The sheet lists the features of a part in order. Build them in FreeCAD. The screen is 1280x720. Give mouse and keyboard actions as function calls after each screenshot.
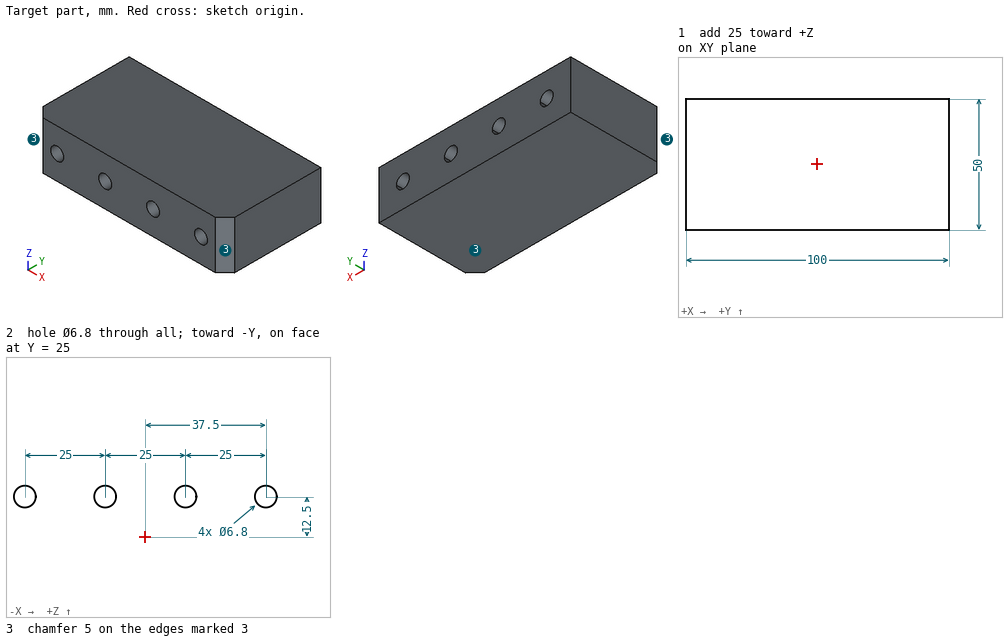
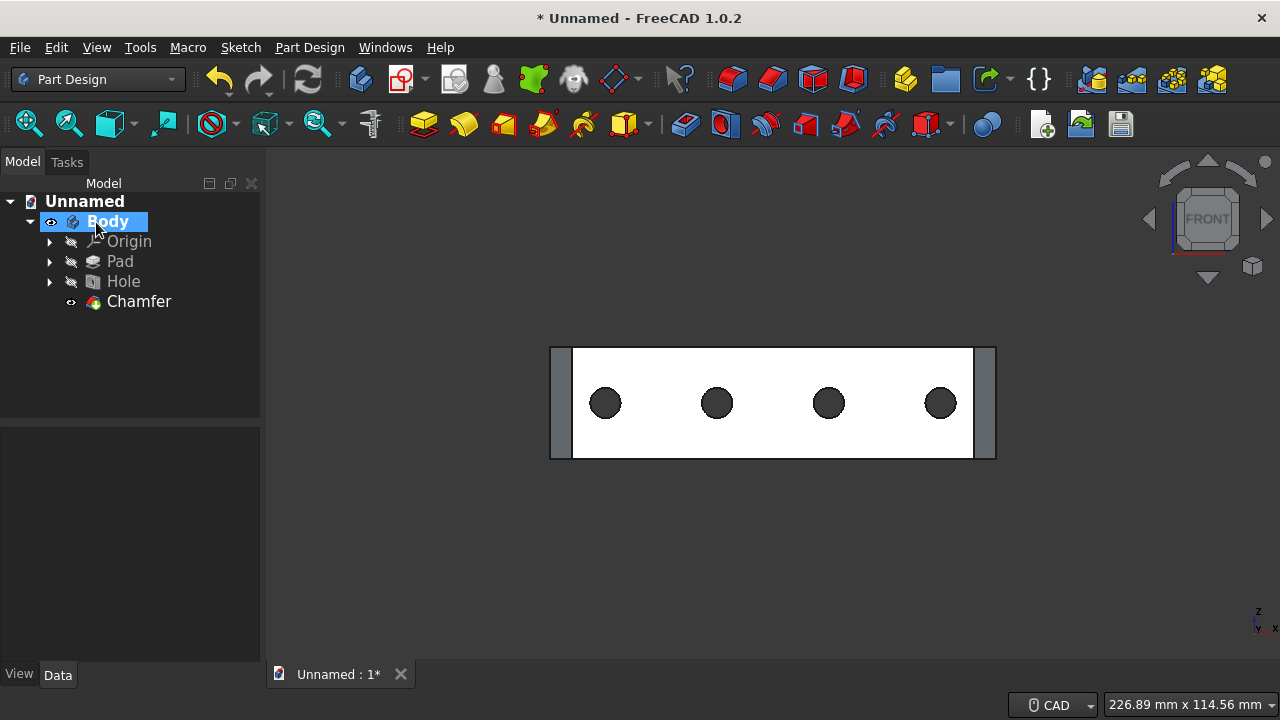
key(0)